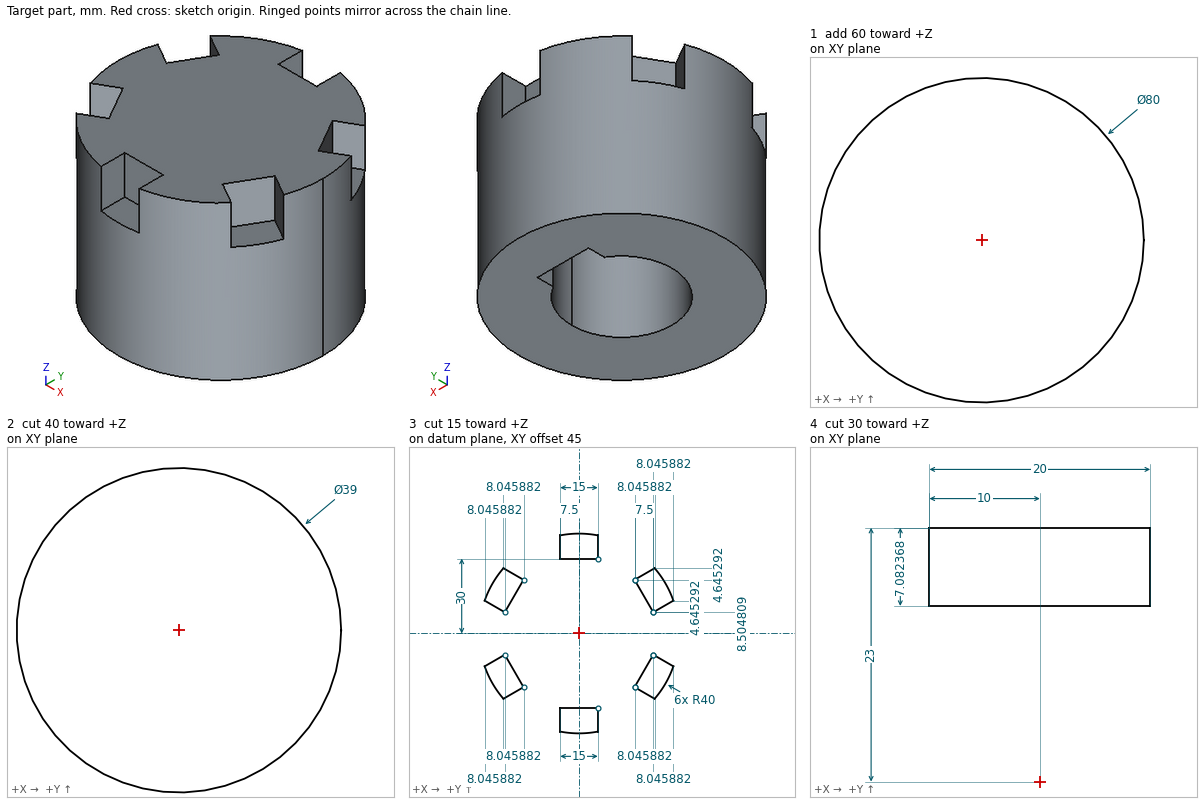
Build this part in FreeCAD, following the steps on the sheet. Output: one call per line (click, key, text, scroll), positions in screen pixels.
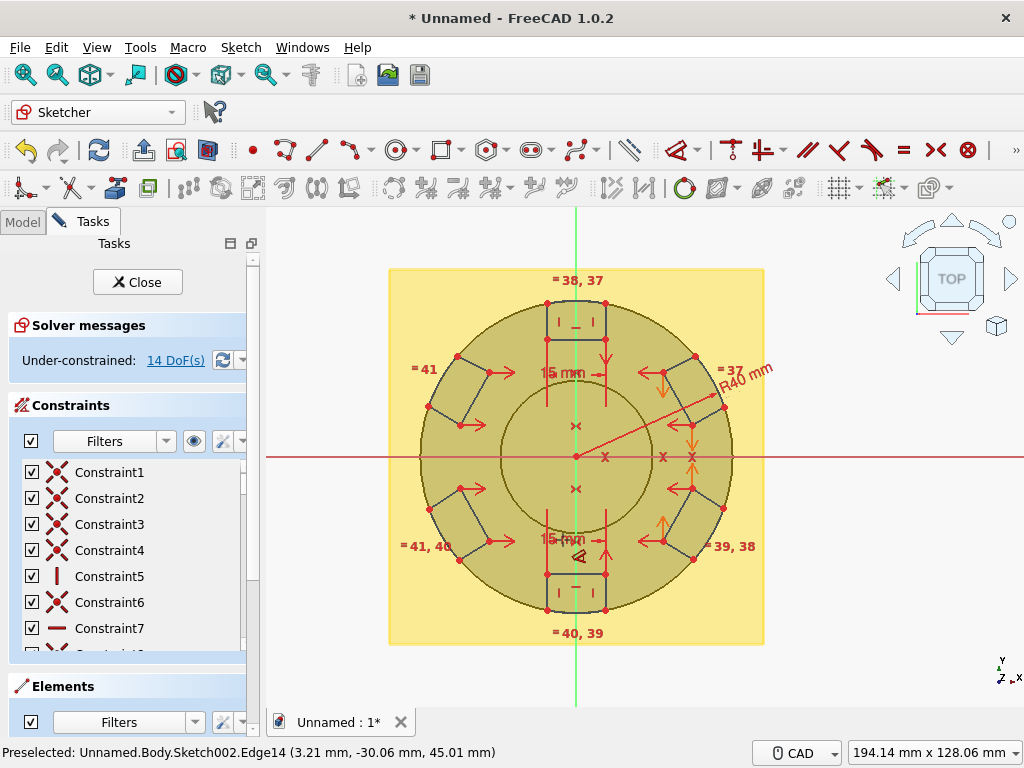
click(547, 340)
click(513, 398)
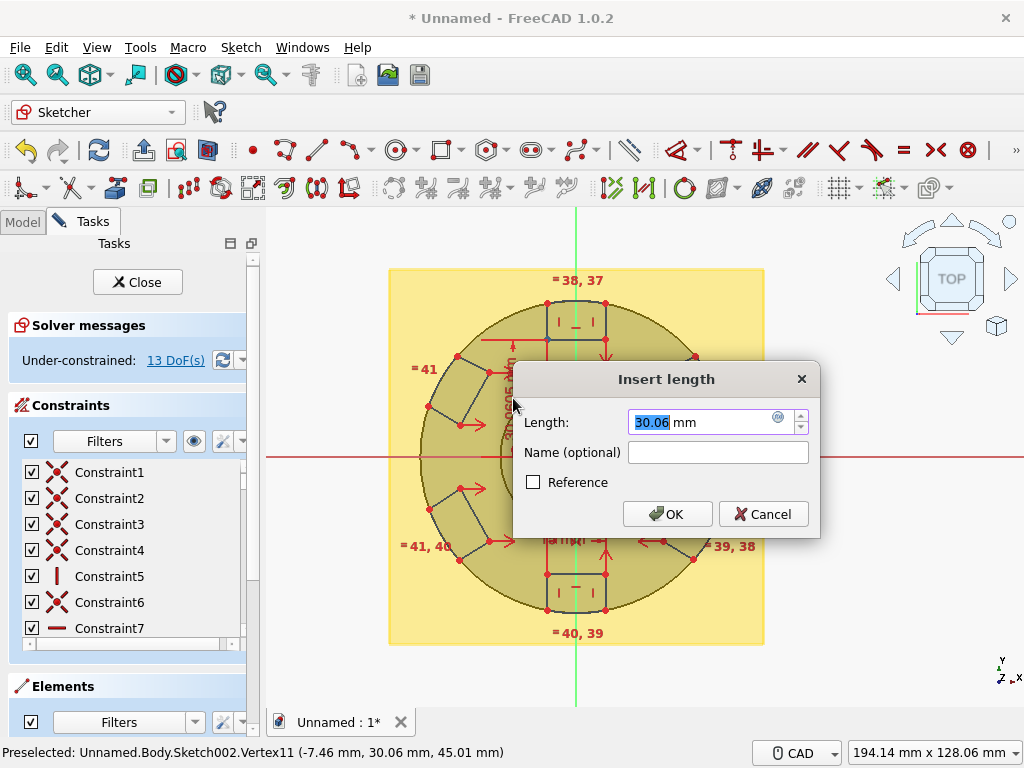
text(30)
key(Return)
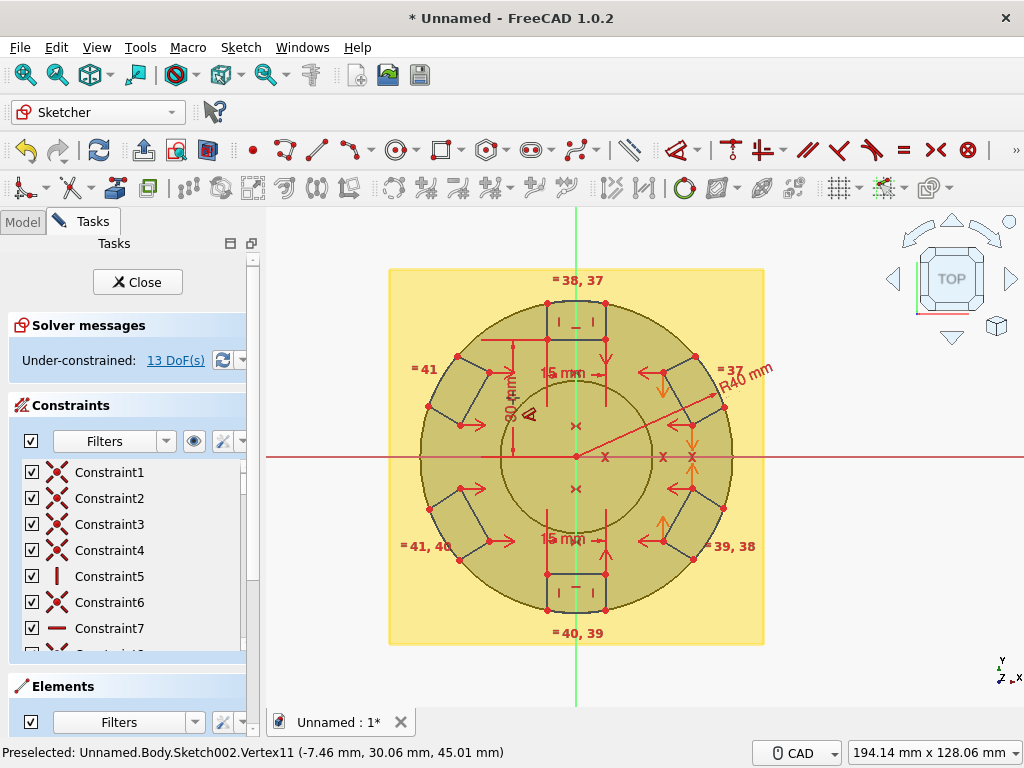
scroll(547, 304, up, 2)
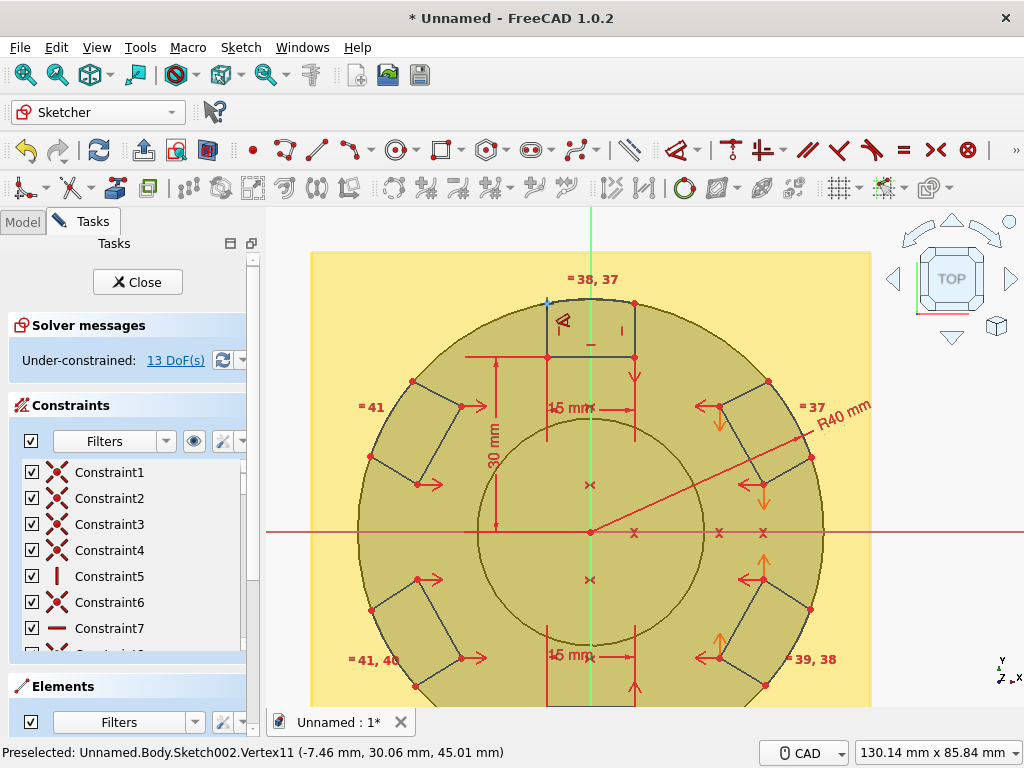
click(547, 303)
click(569, 269)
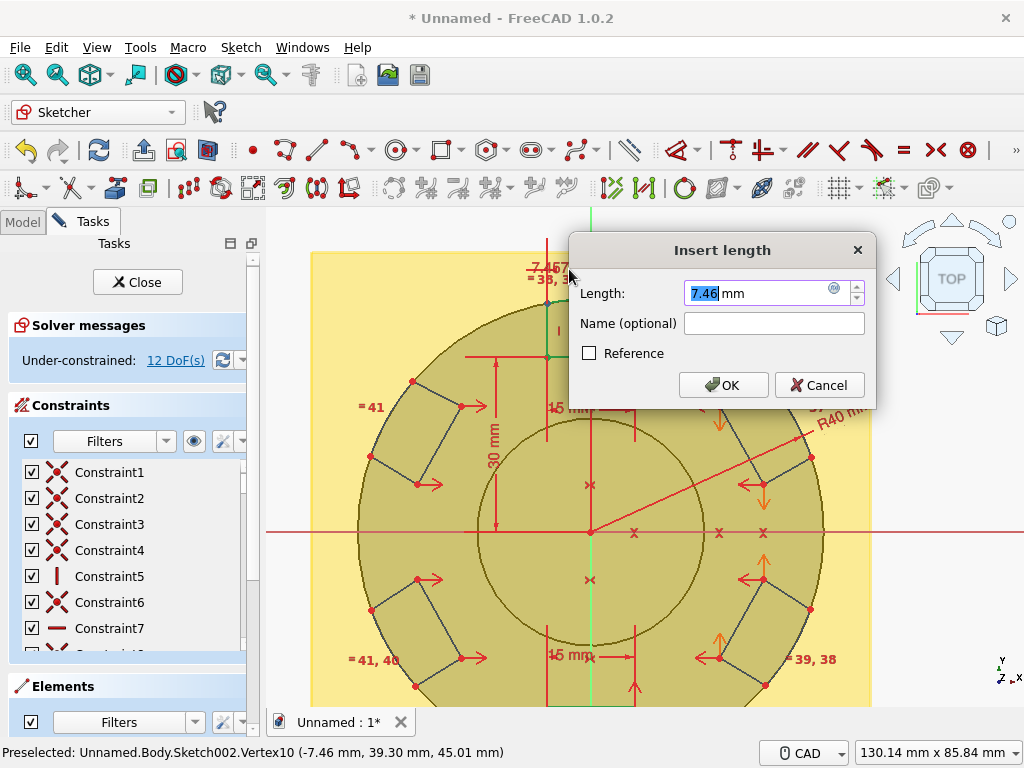
text(7.5)
key(Return)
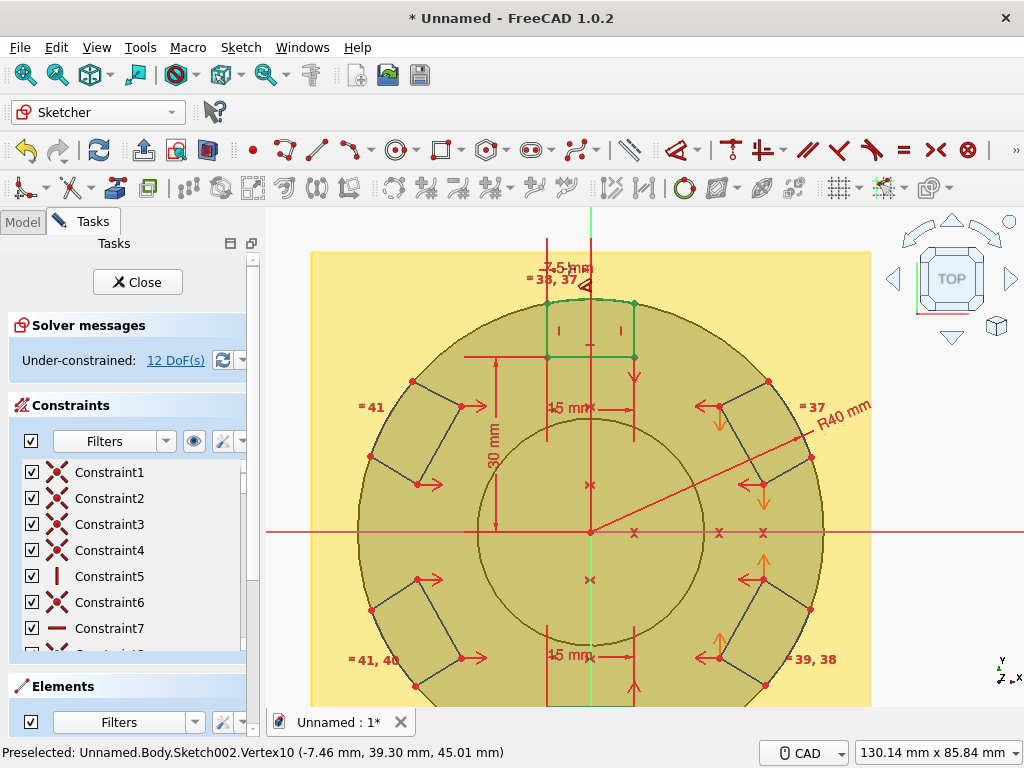
click(733, 430)
click(742, 372)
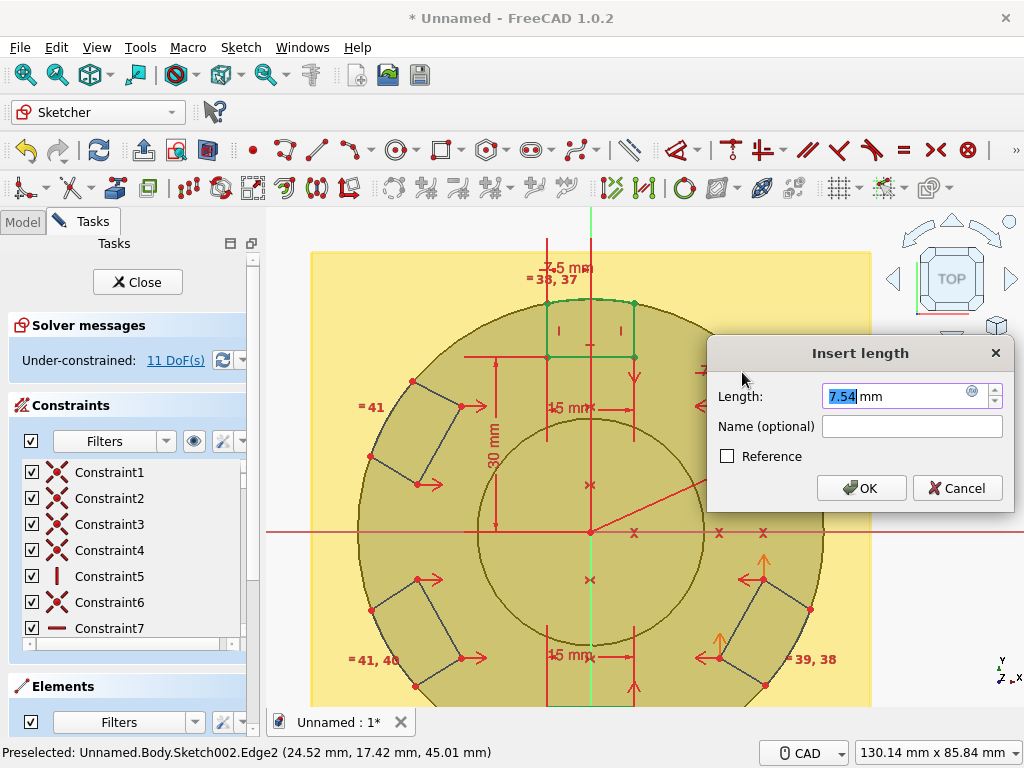
text(7.5)
key(Return)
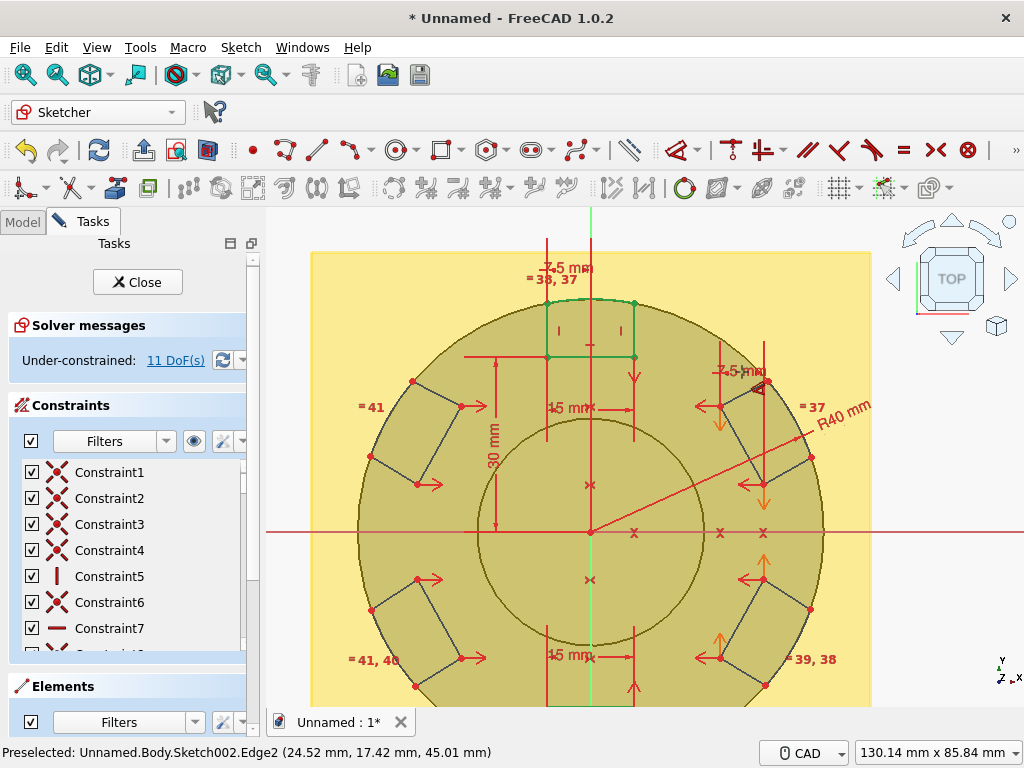
click(764, 485)
click(798, 508)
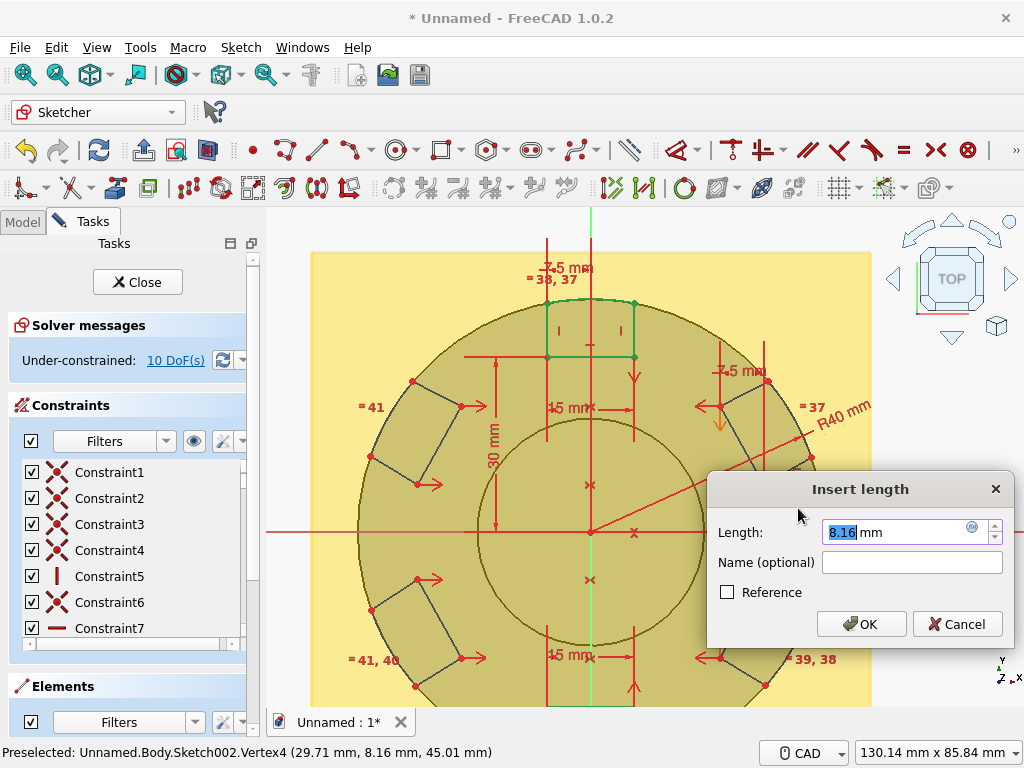
text(8.504809)
key(Return)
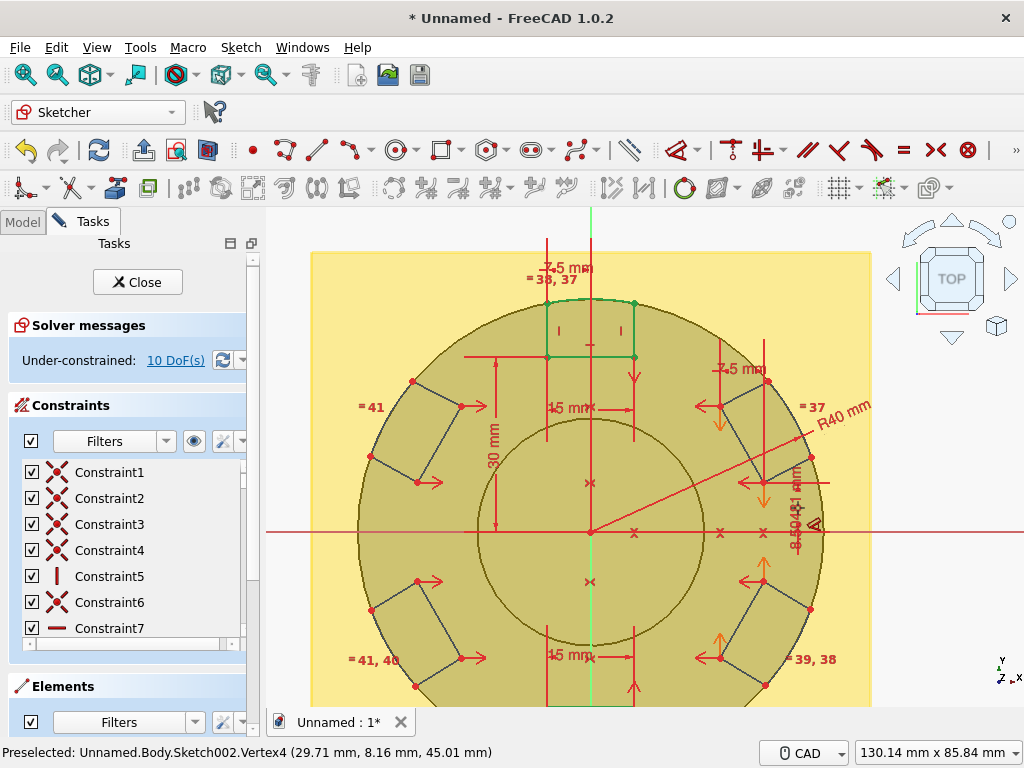
click(754, 389)
click(744, 348)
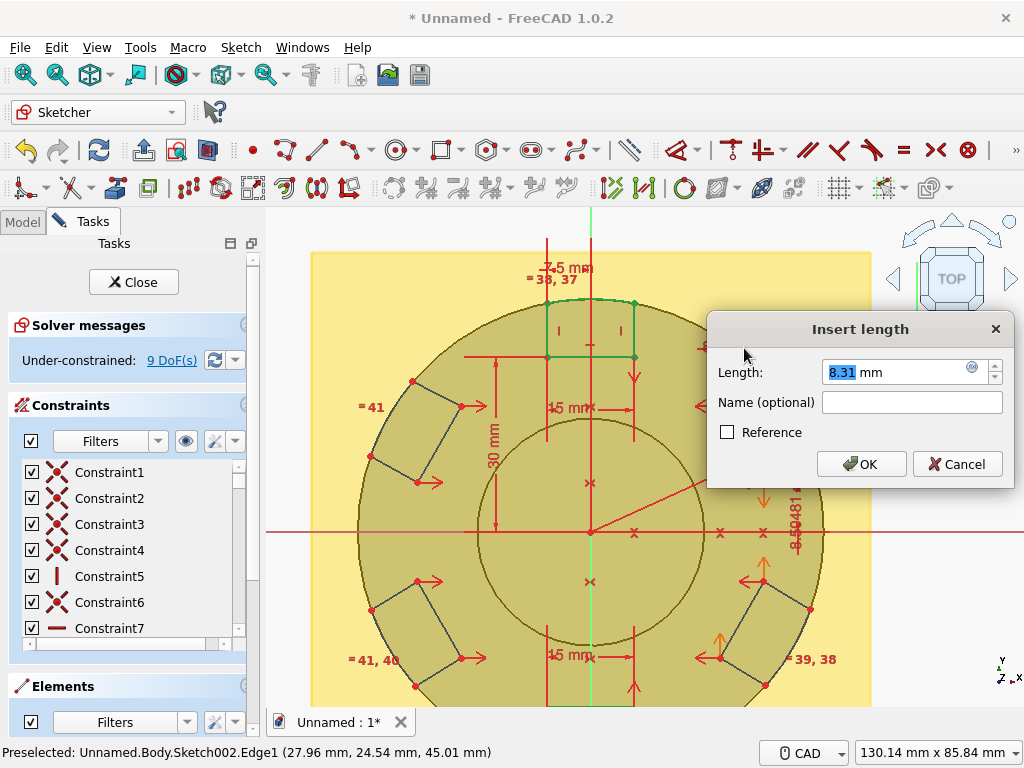
text(8.045882)
key(Return)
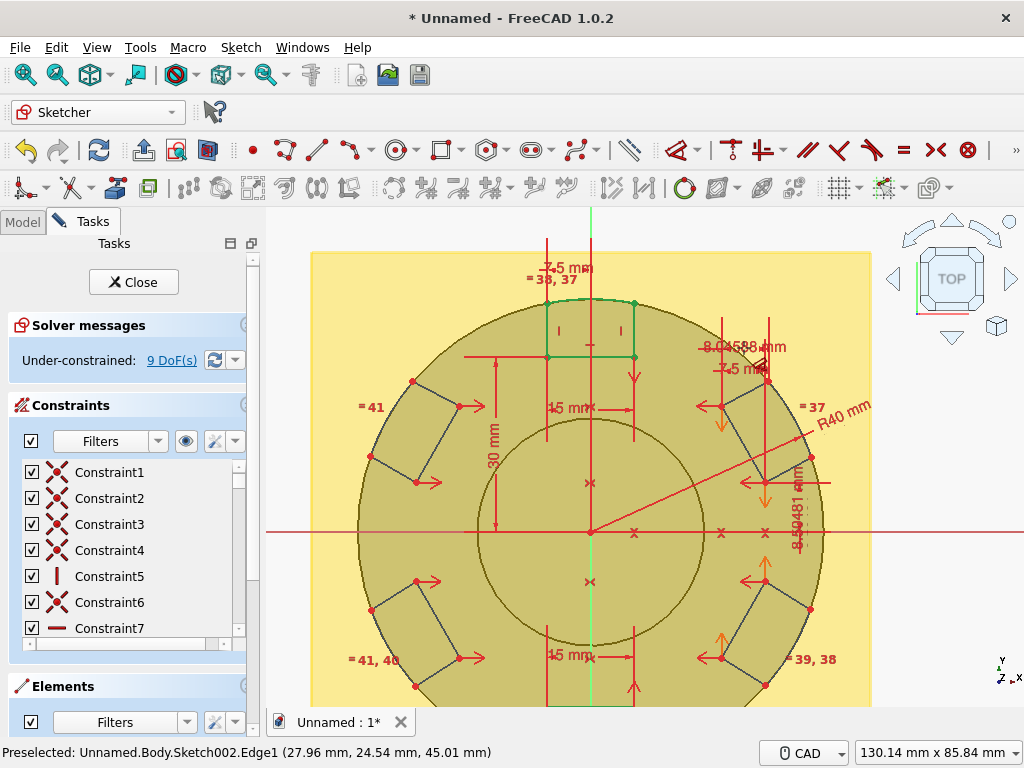
scroll(755, 389, up, 2)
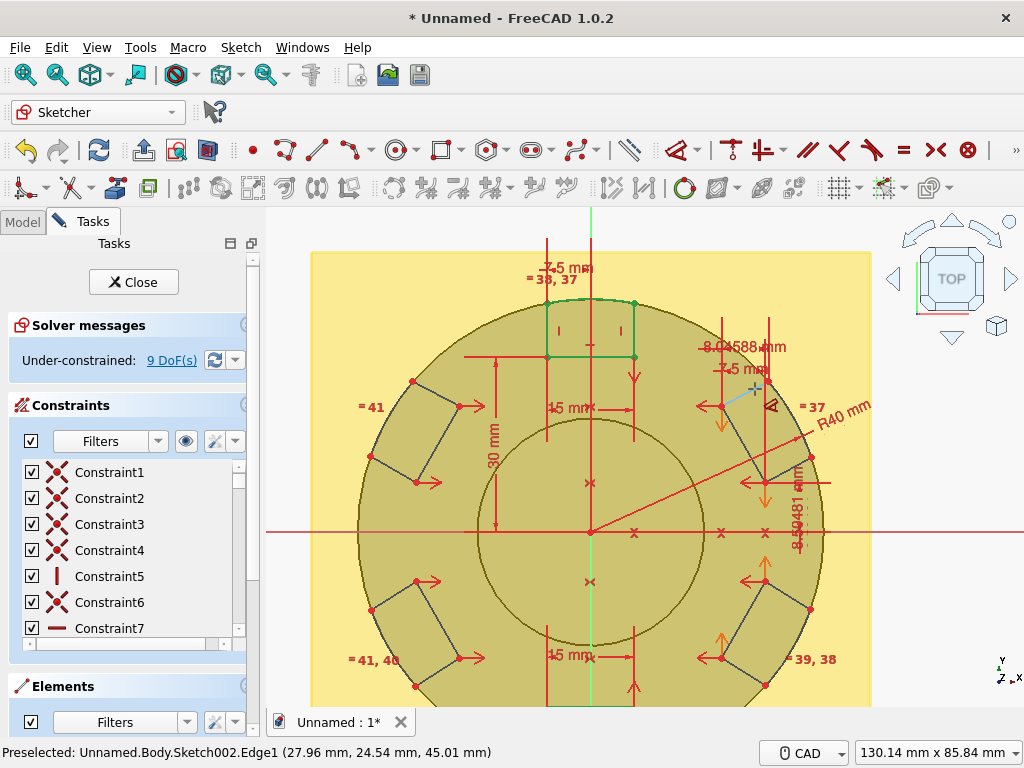
click(754, 389)
click(809, 396)